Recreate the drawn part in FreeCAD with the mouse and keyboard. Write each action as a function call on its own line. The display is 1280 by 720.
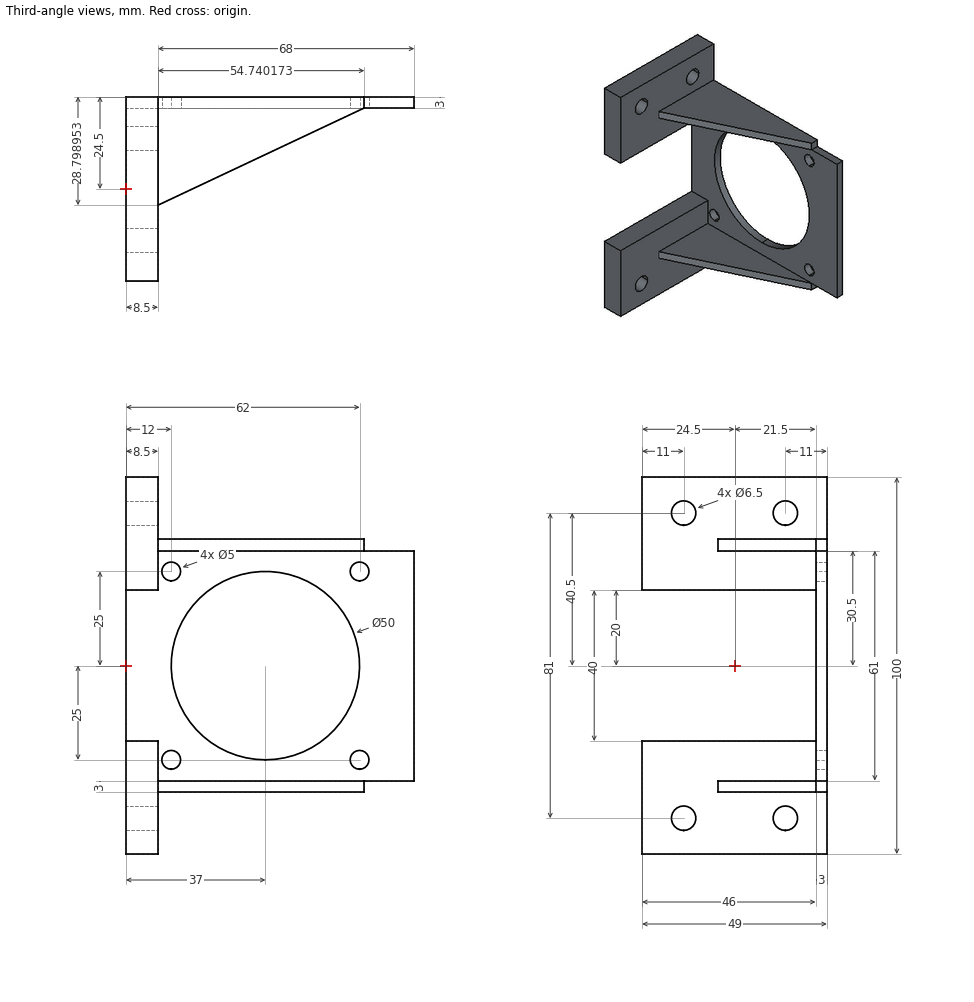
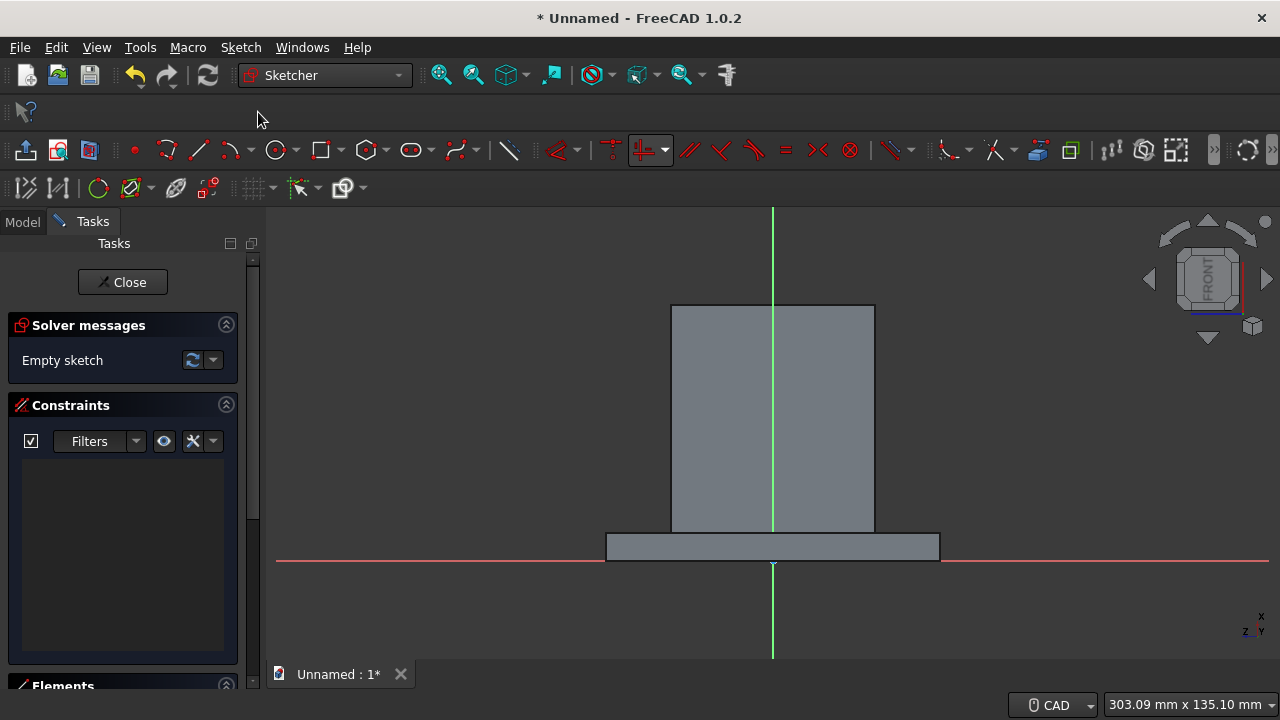
click(276, 150)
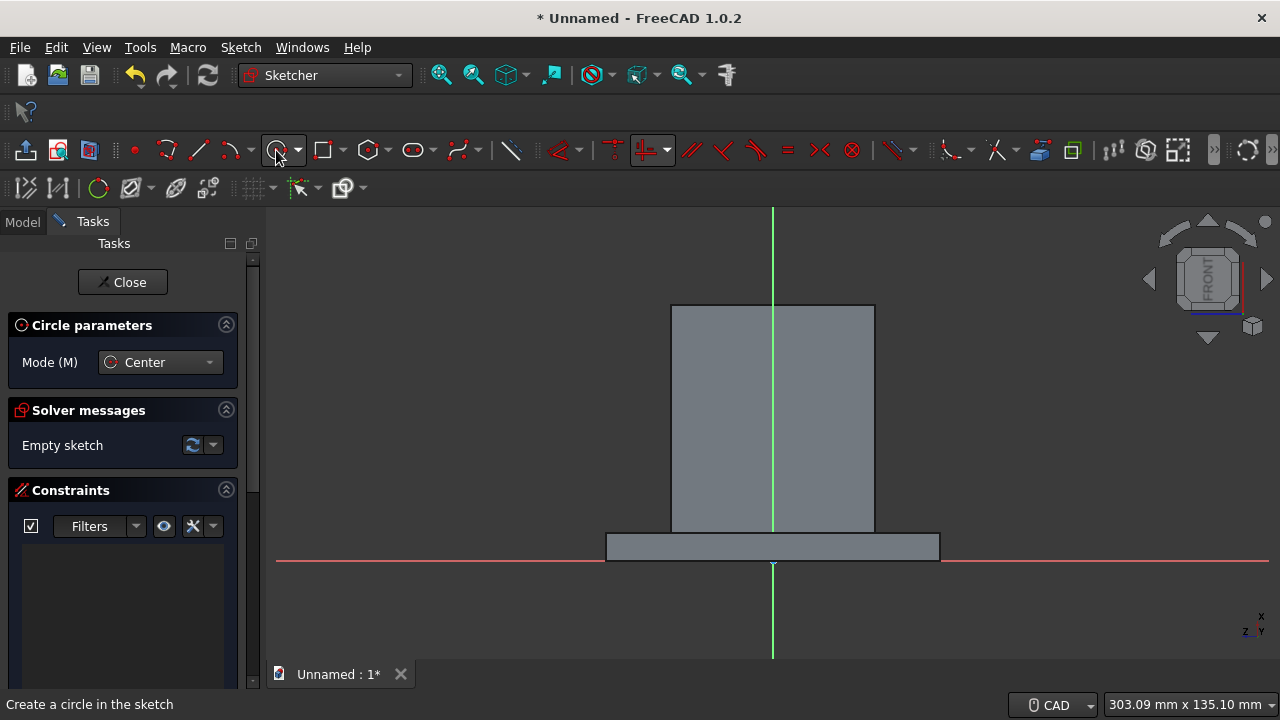
click(773, 437)
click(832, 378)
key(Escape)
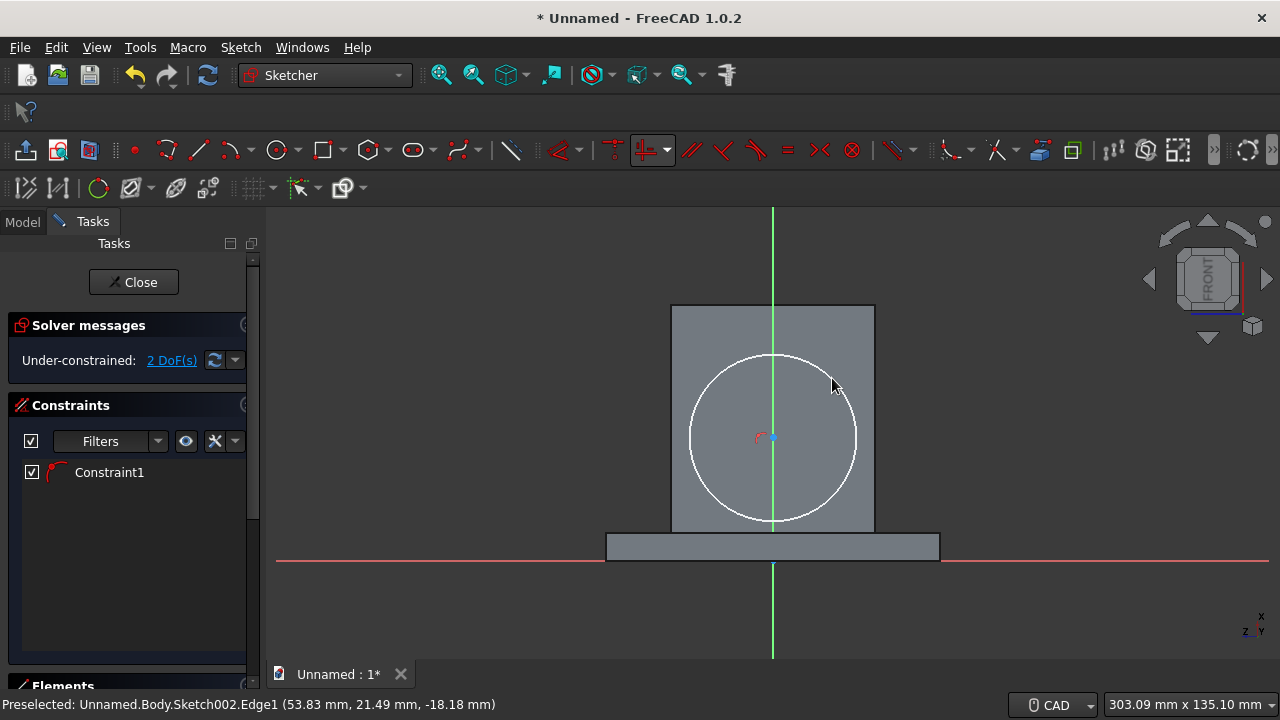
click(558, 150)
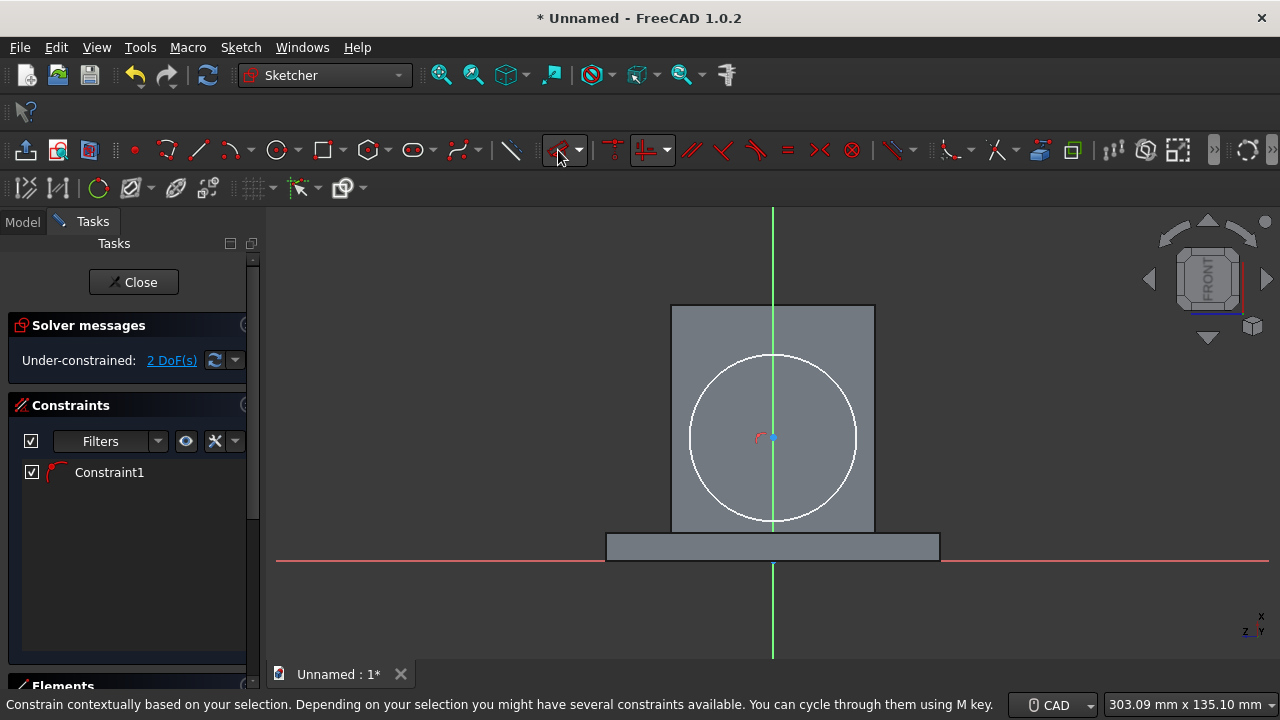
click(832, 379)
click(855, 356)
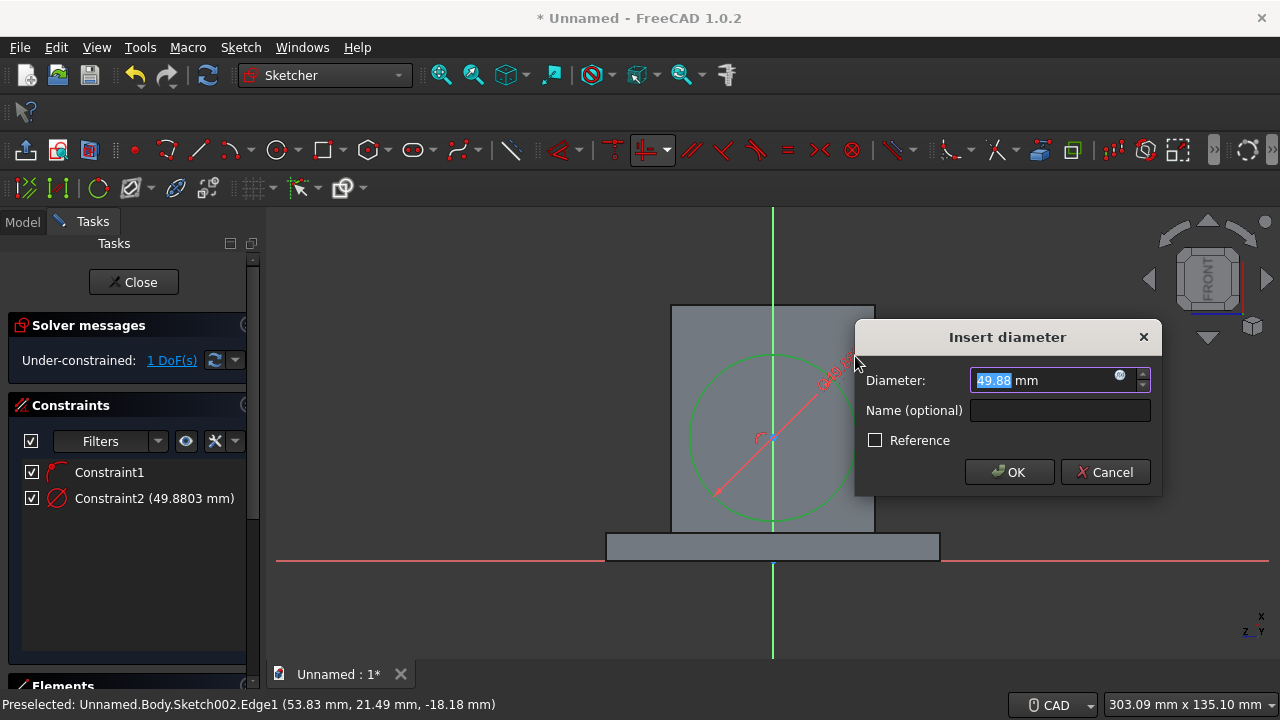
text(50)
key(Return)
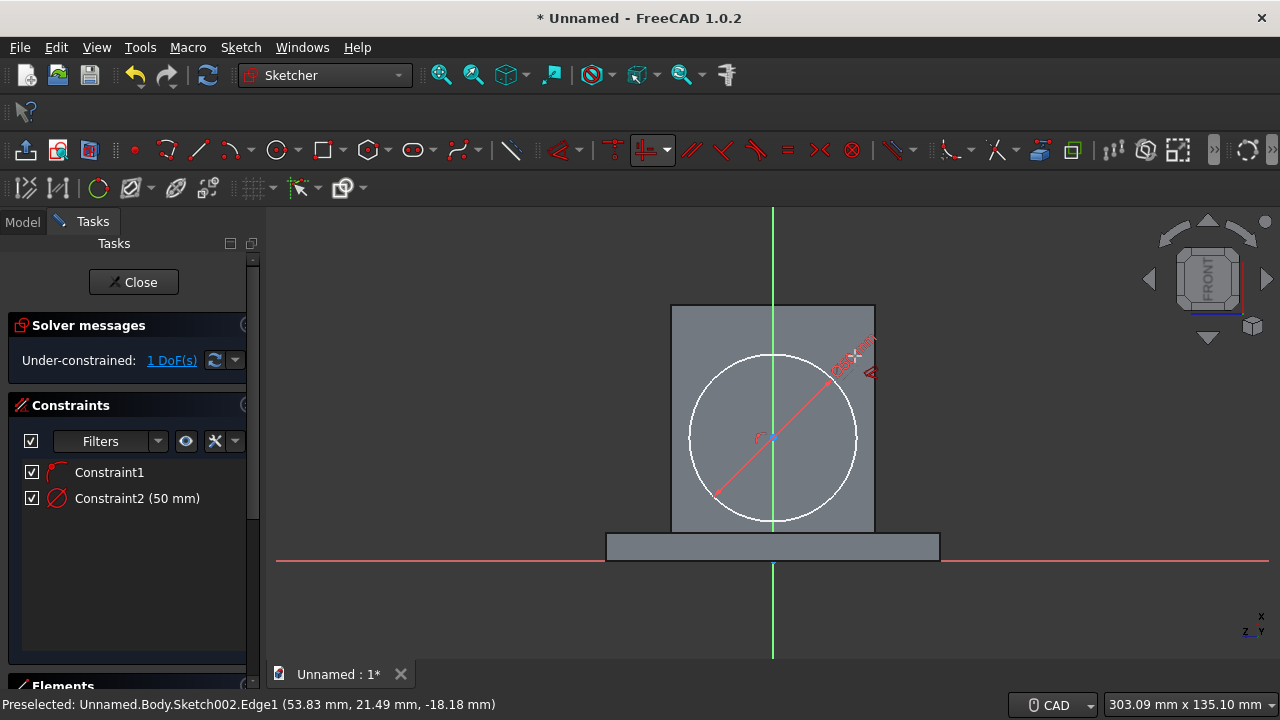
click(773, 438)
click(807, 499)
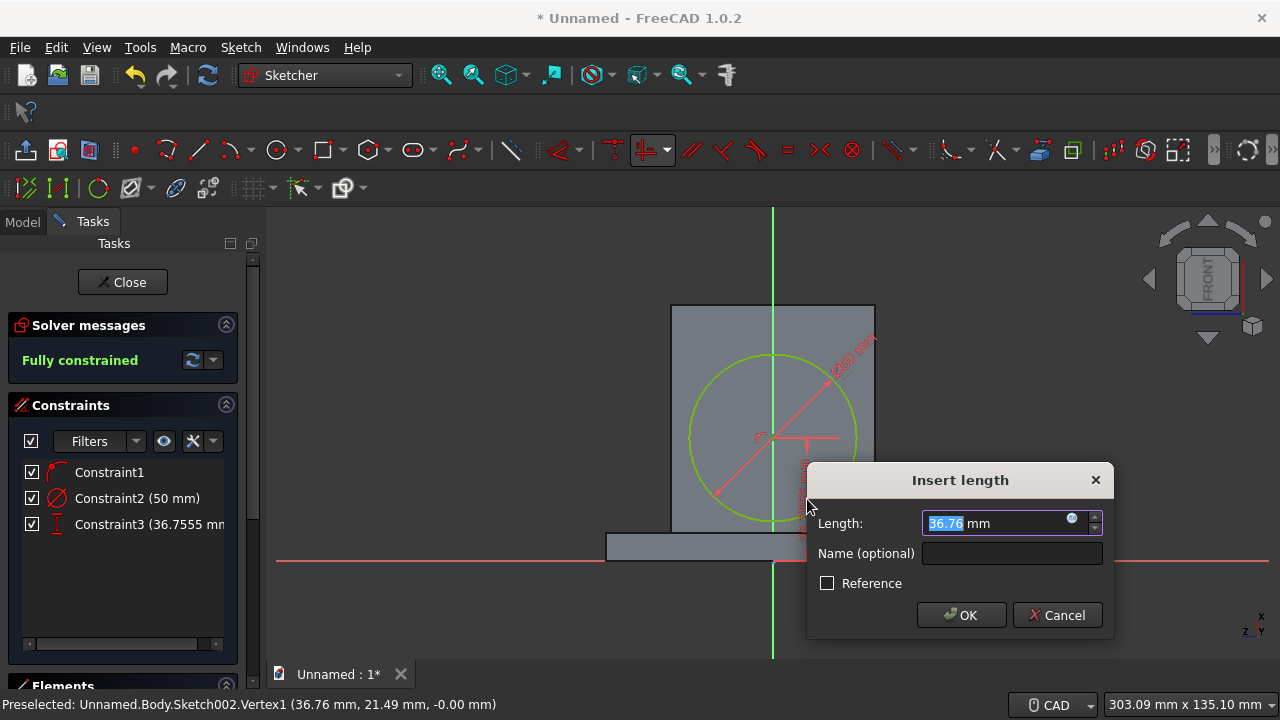
text(37)
key(Return)
key(Escape)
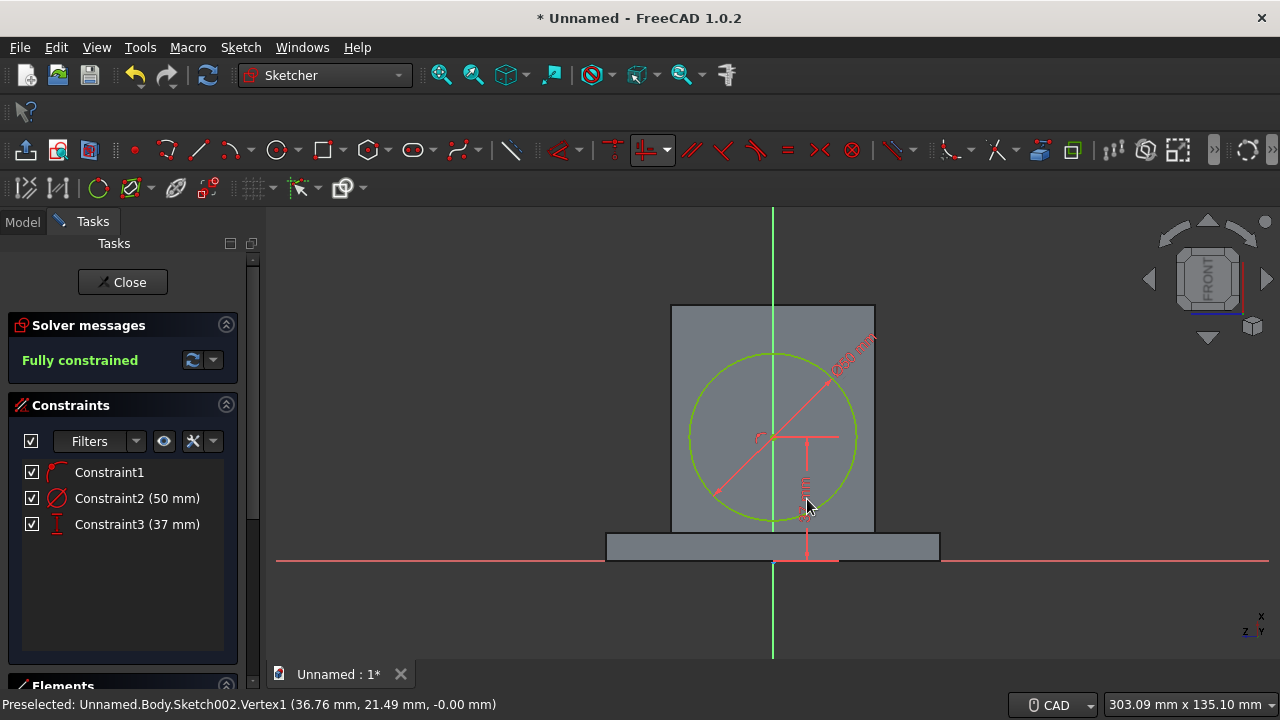
click(123, 282)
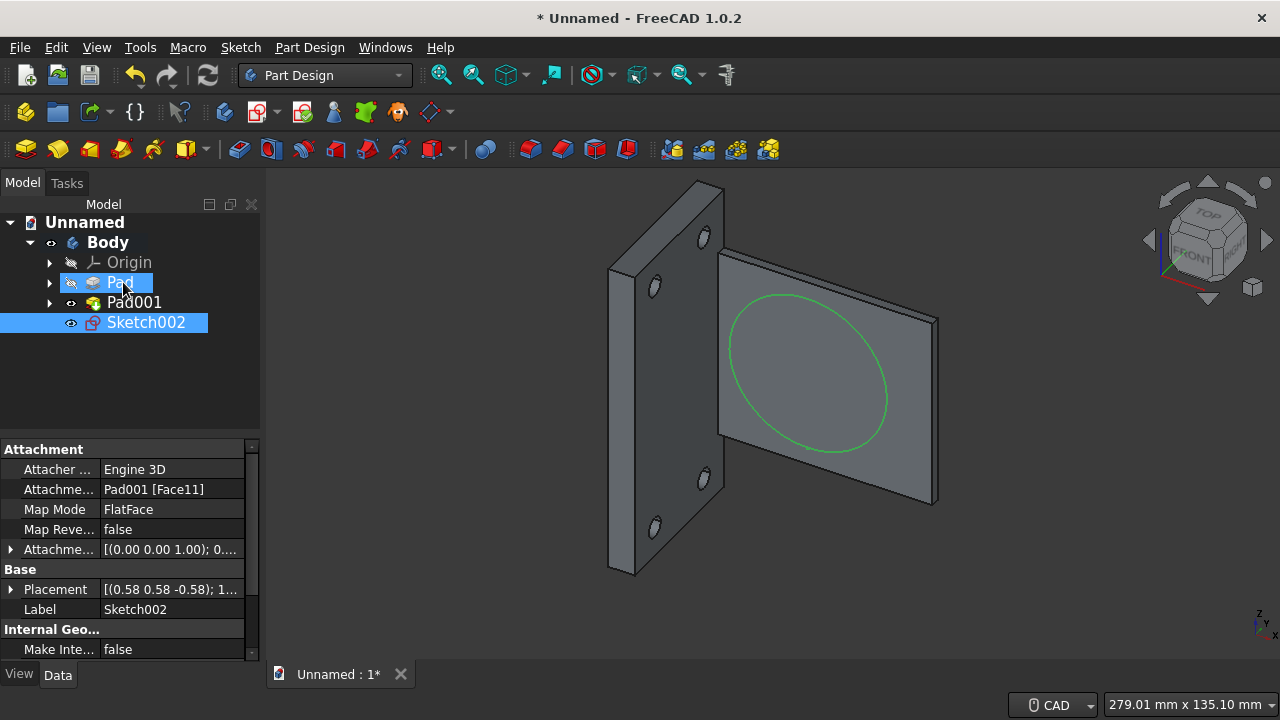
click(240, 150)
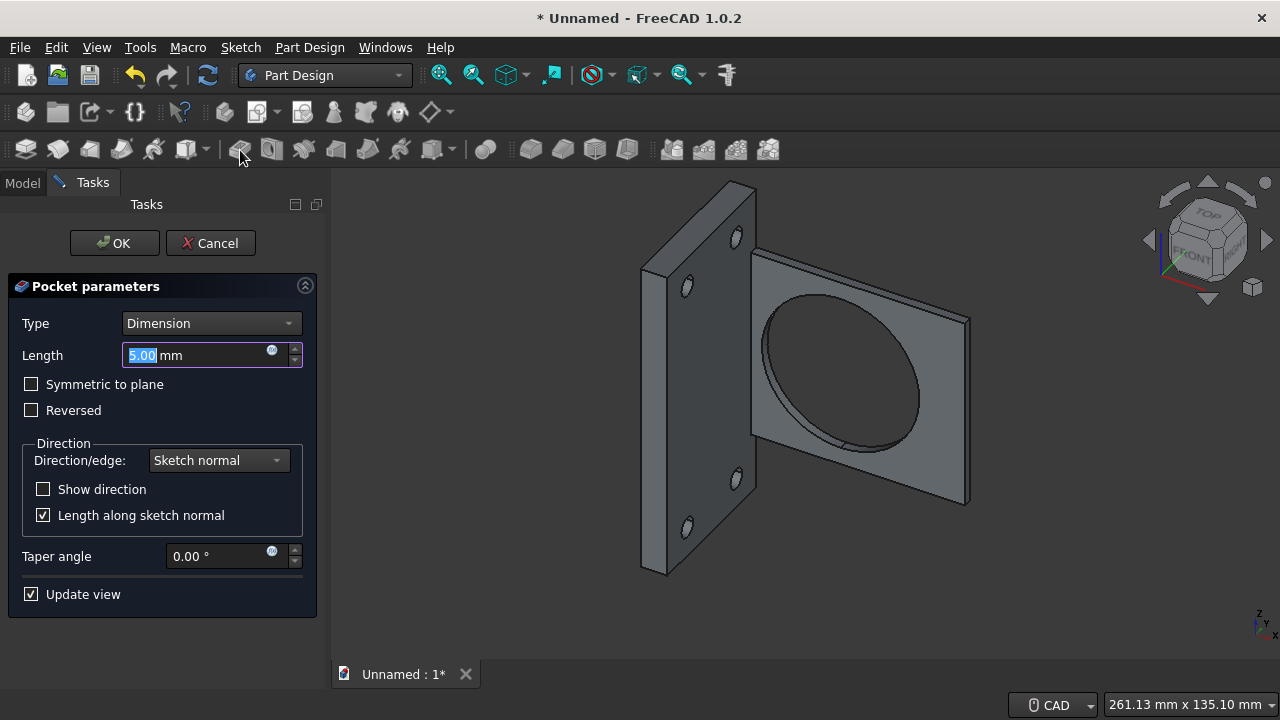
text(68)
key(Tab)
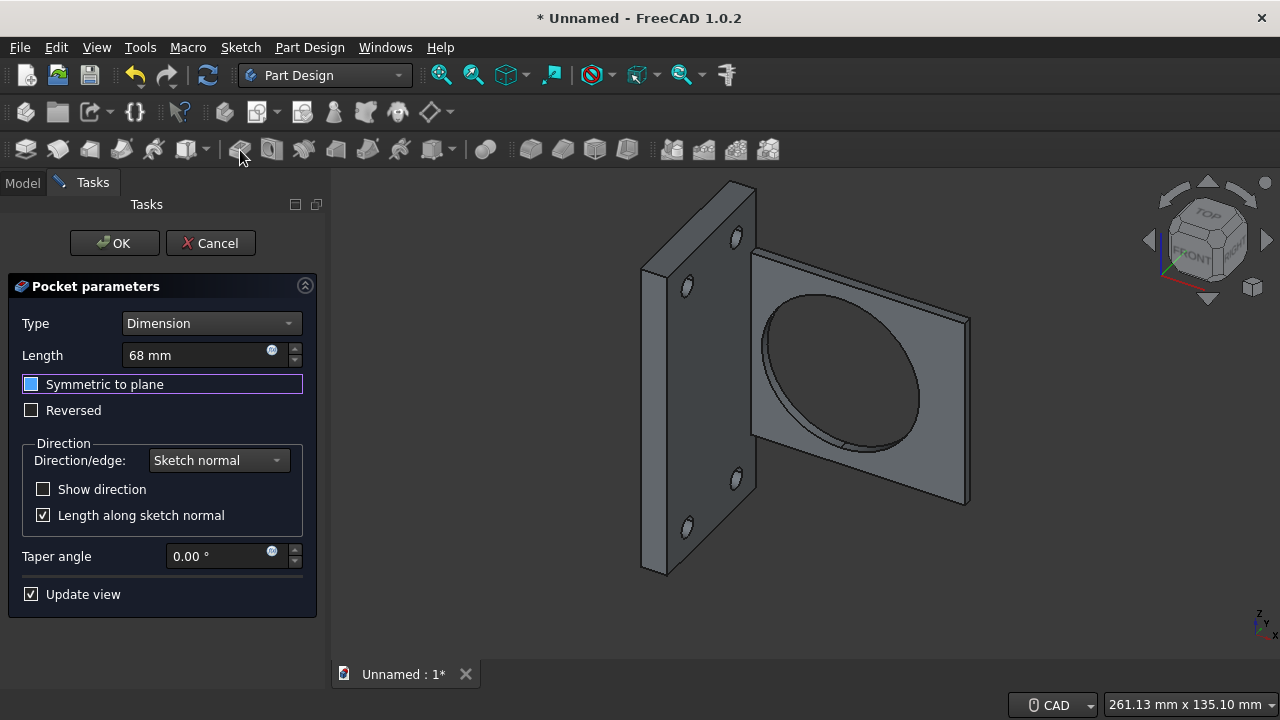
click(115, 243)